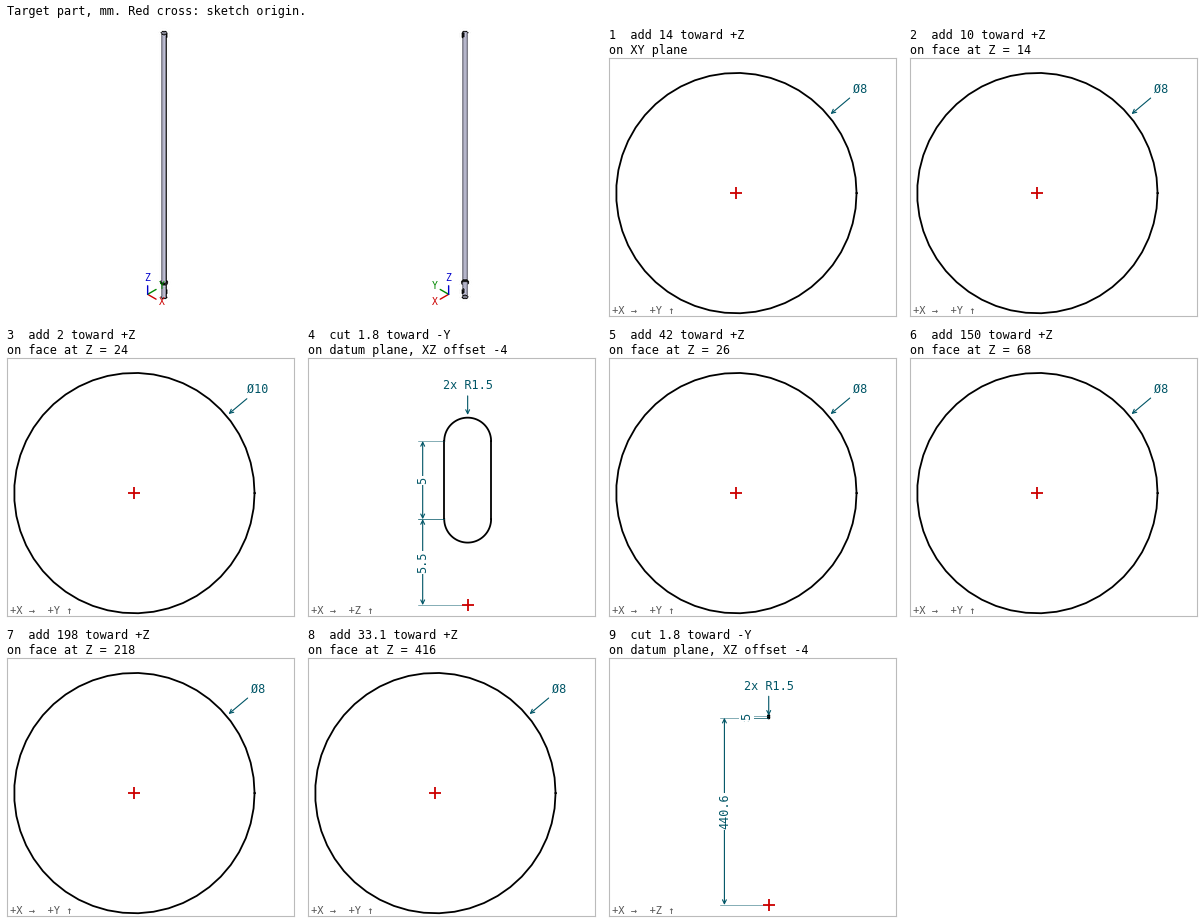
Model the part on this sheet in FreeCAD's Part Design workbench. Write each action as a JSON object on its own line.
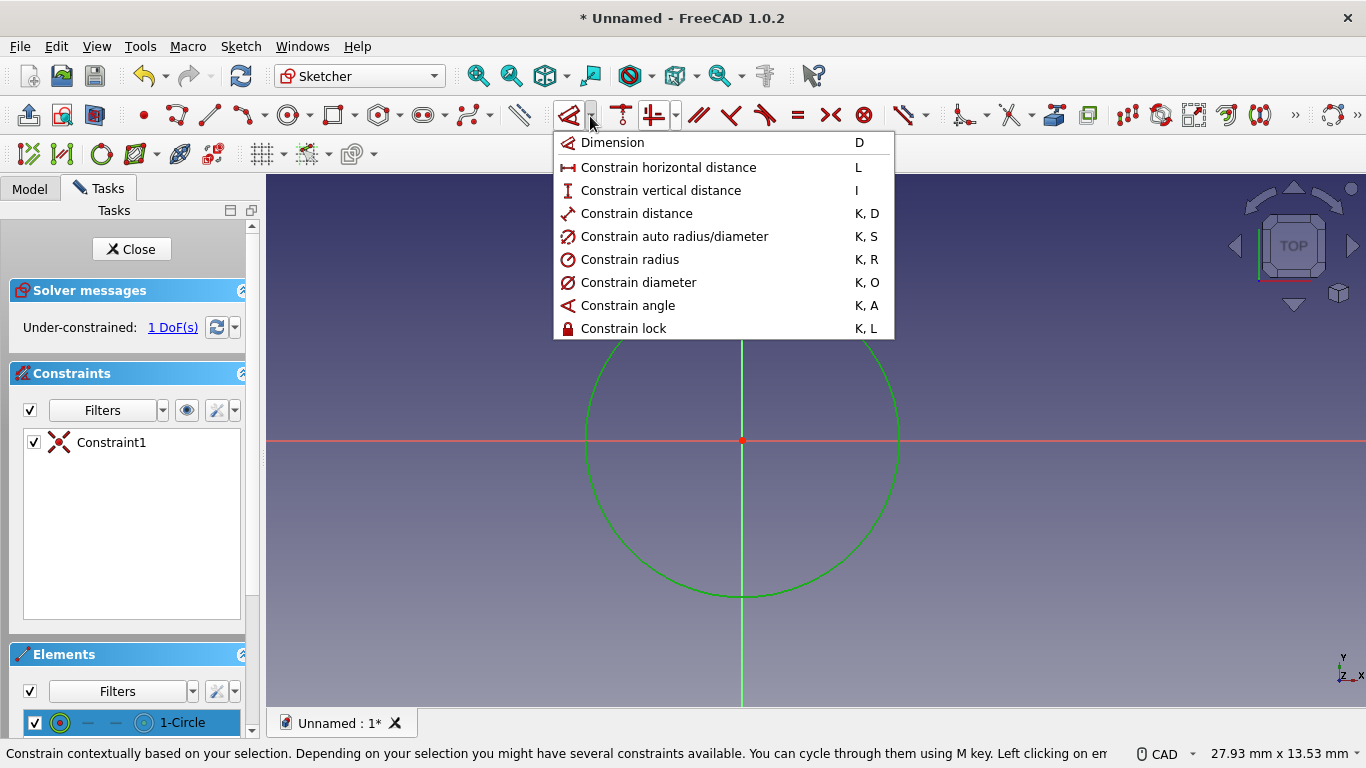
{"action": "left_click", "coordinate": [724, 282]}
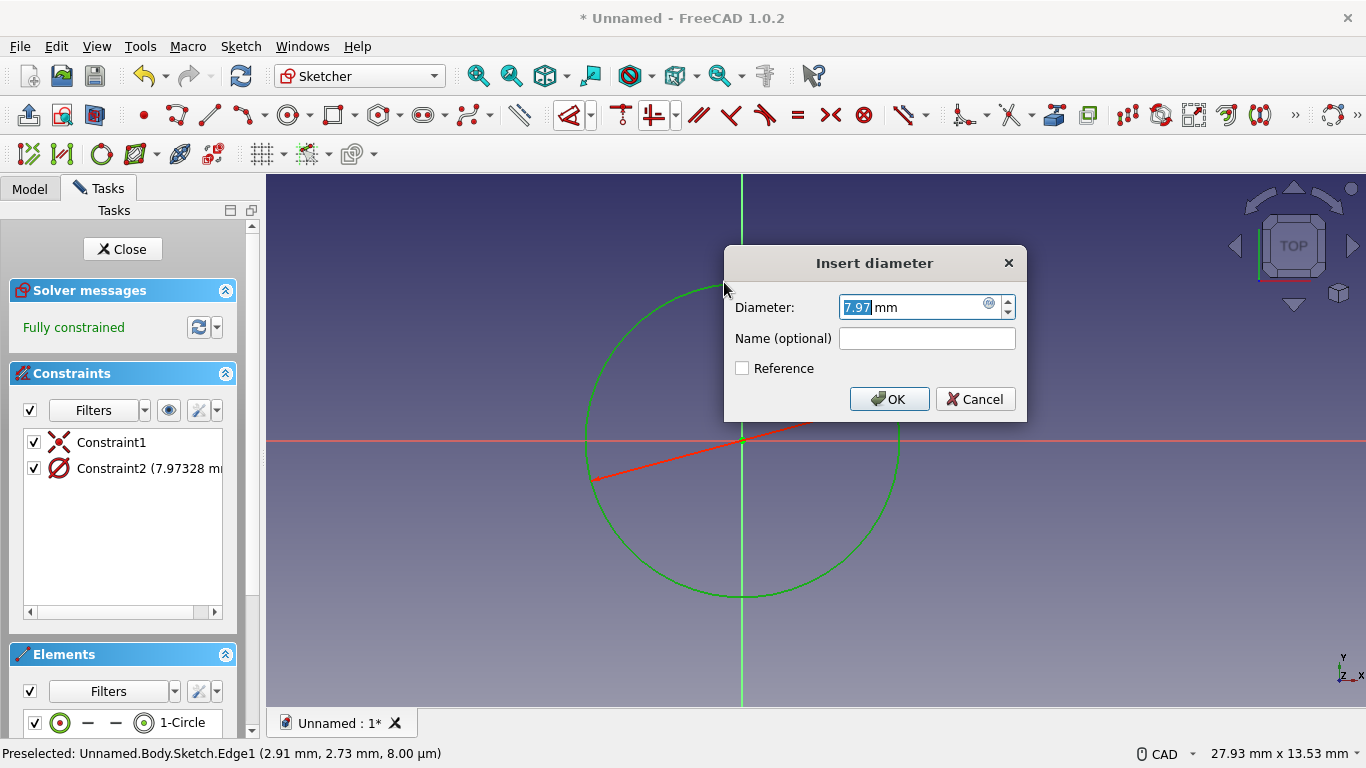
{"action": "type", "text": "8"}
{"action": "key", "text": "Return"}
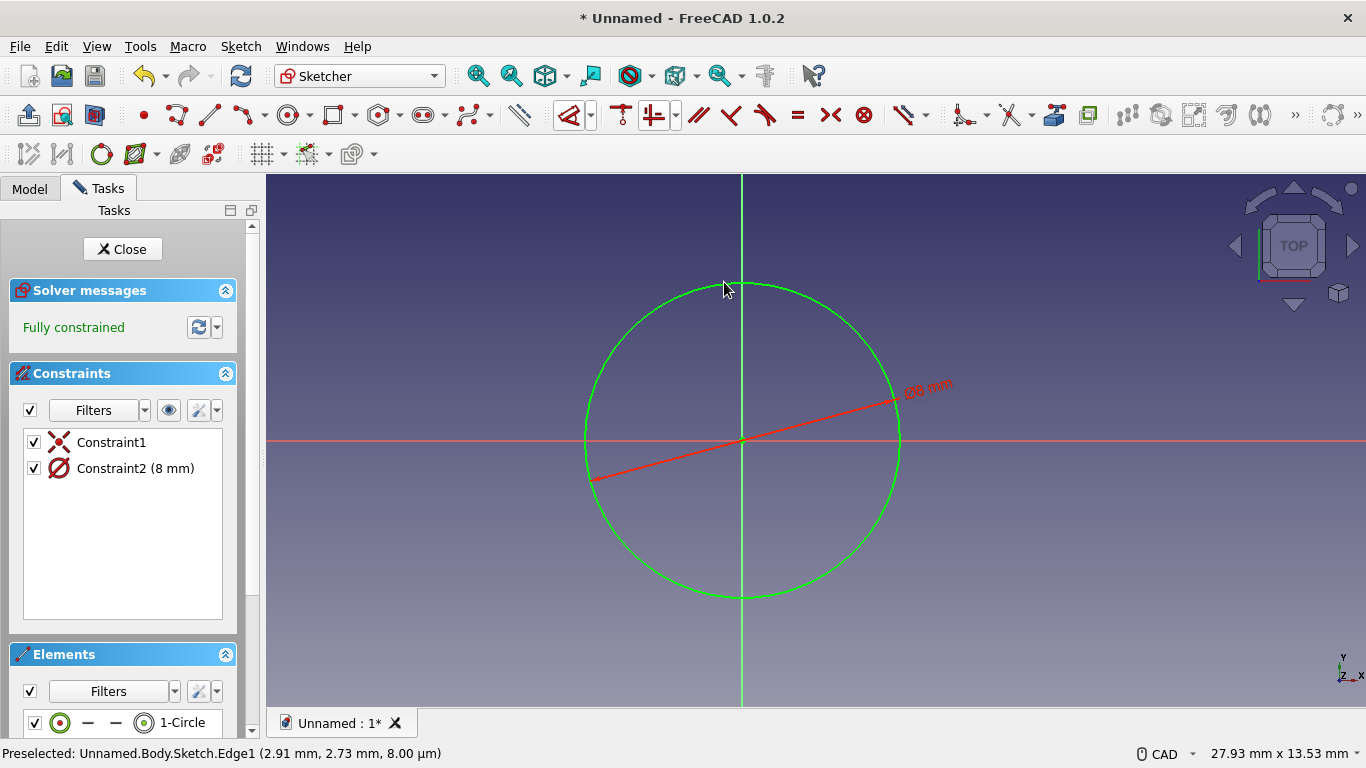
{"action": "left_click", "coordinate": [123, 249]}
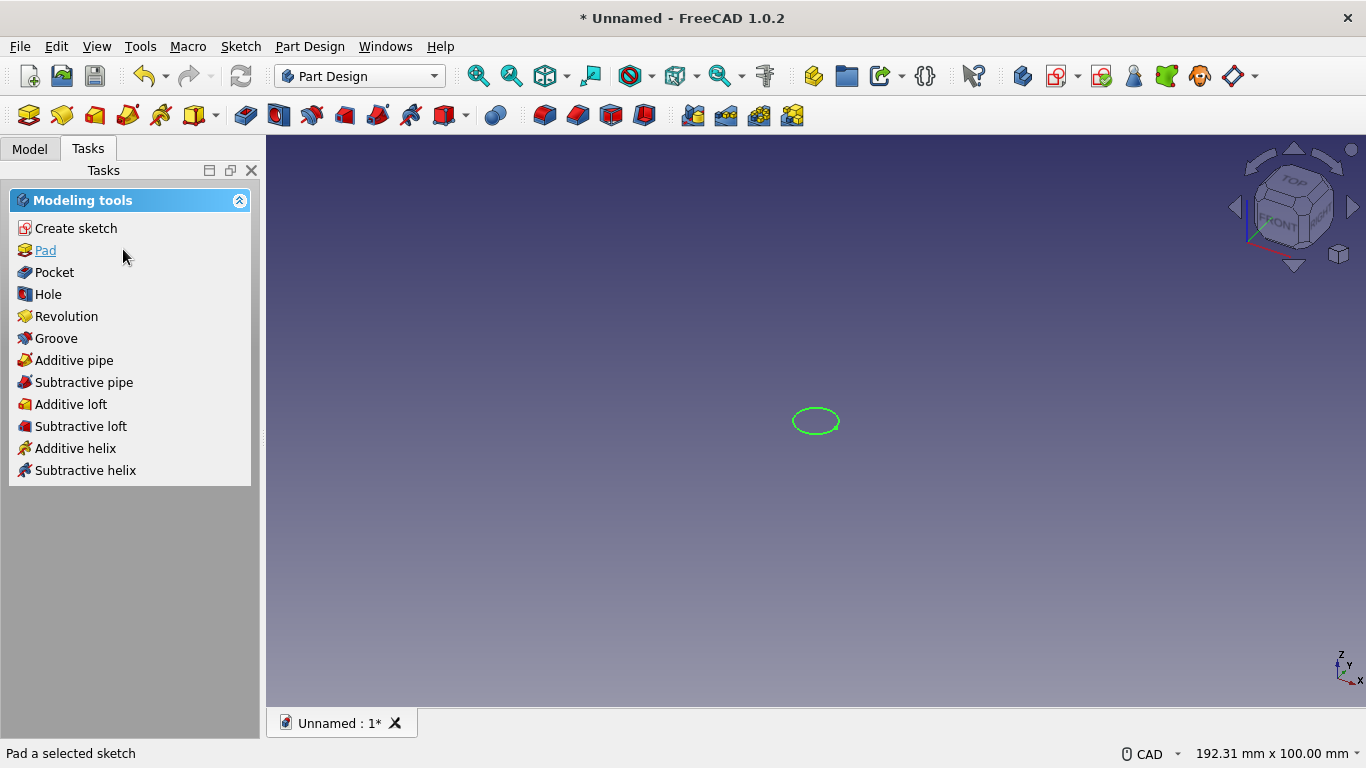
{"action": "left_click", "coordinate": [29, 116]}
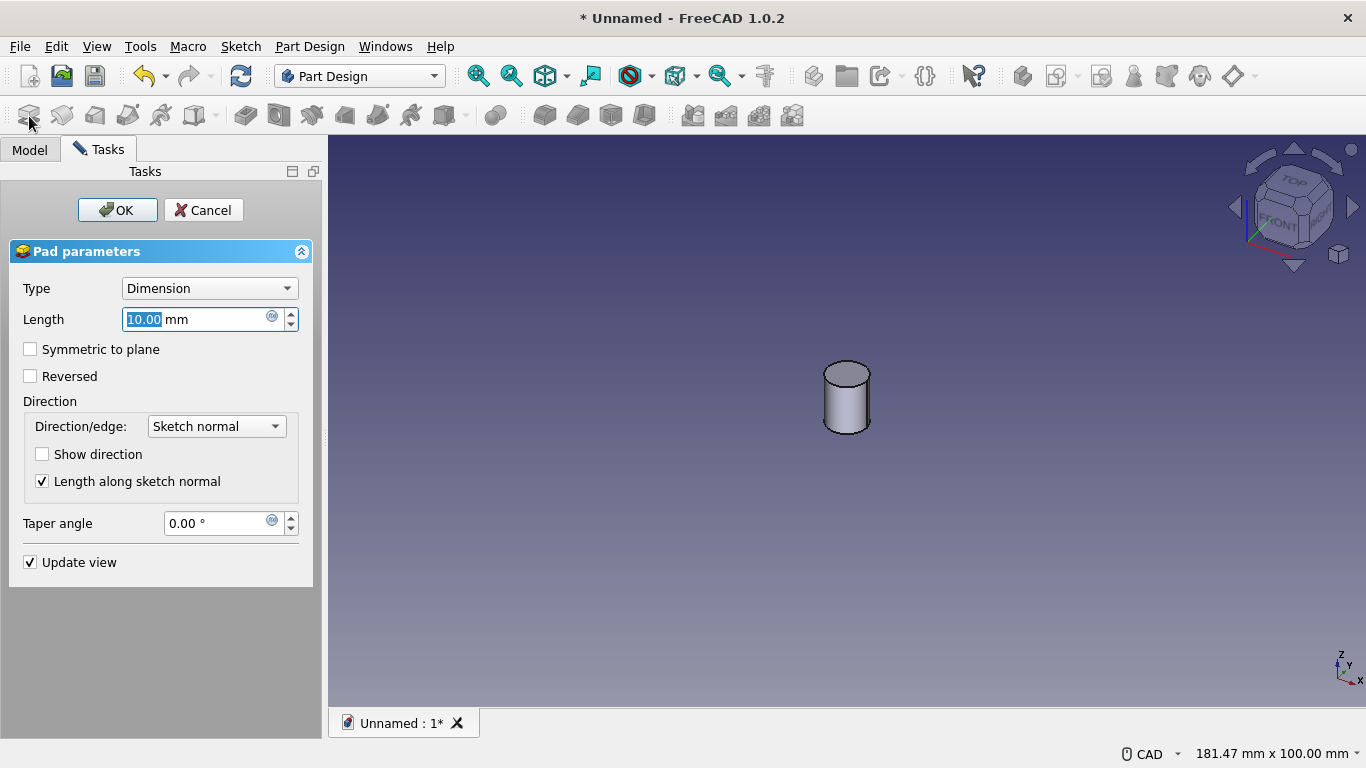
{"action": "type", "text": "14"}
{"action": "key", "text": "Tab"}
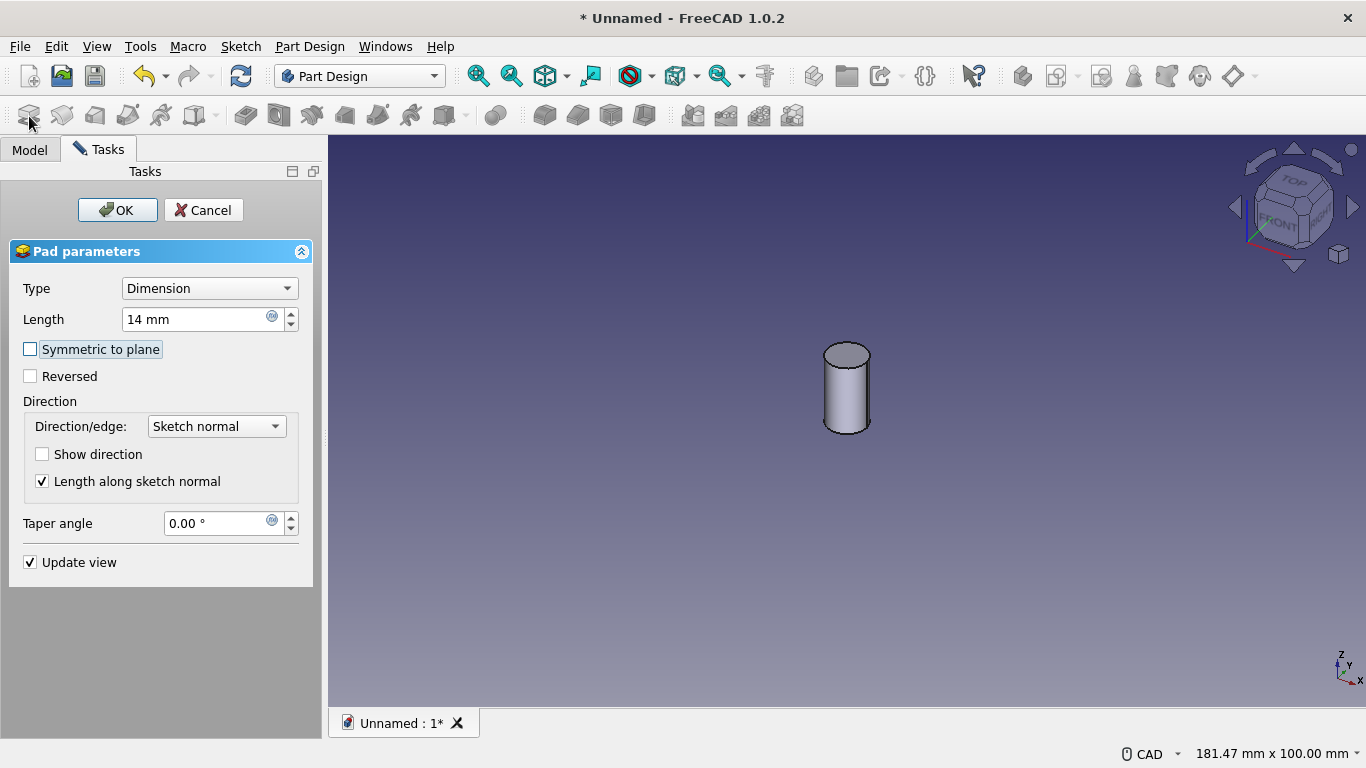
{"action": "left_click", "coordinate": [118, 210]}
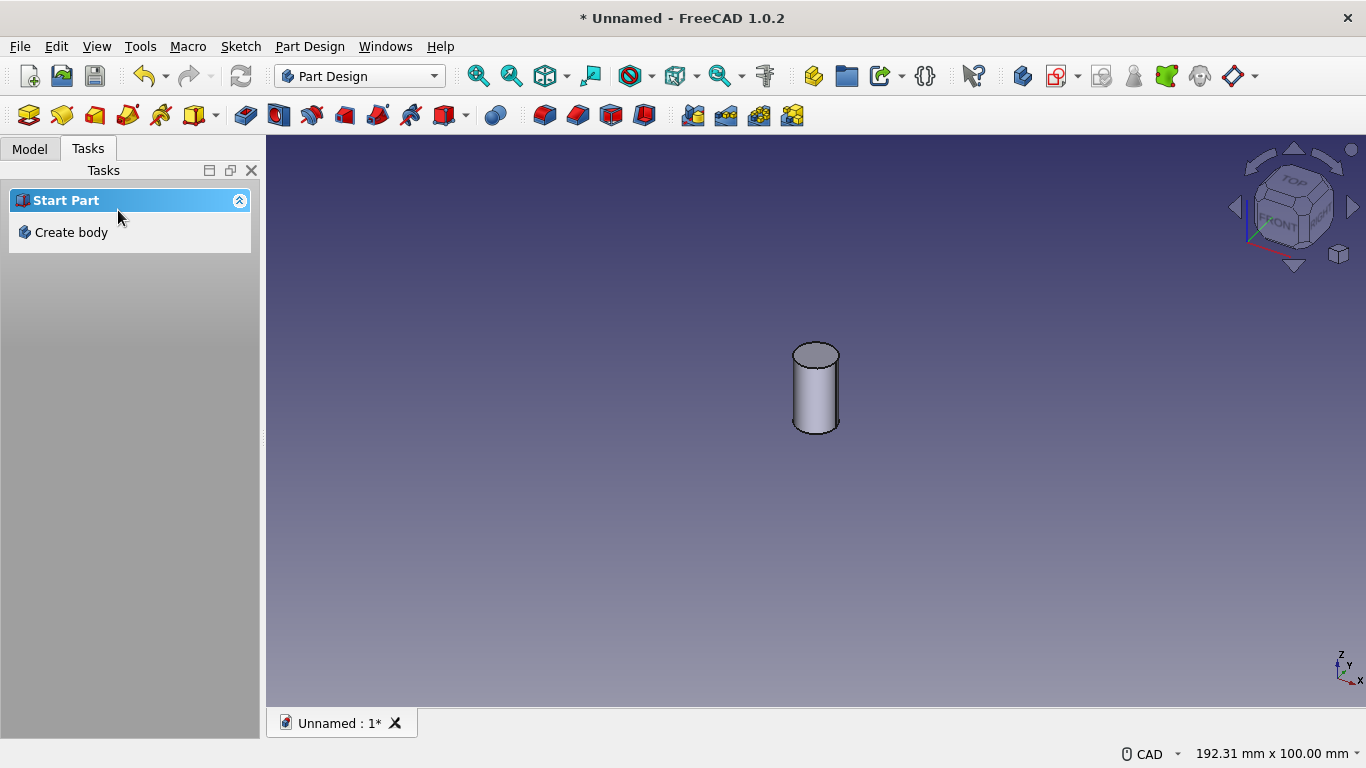
{"action": "left_click", "coordinate": [479, 76]}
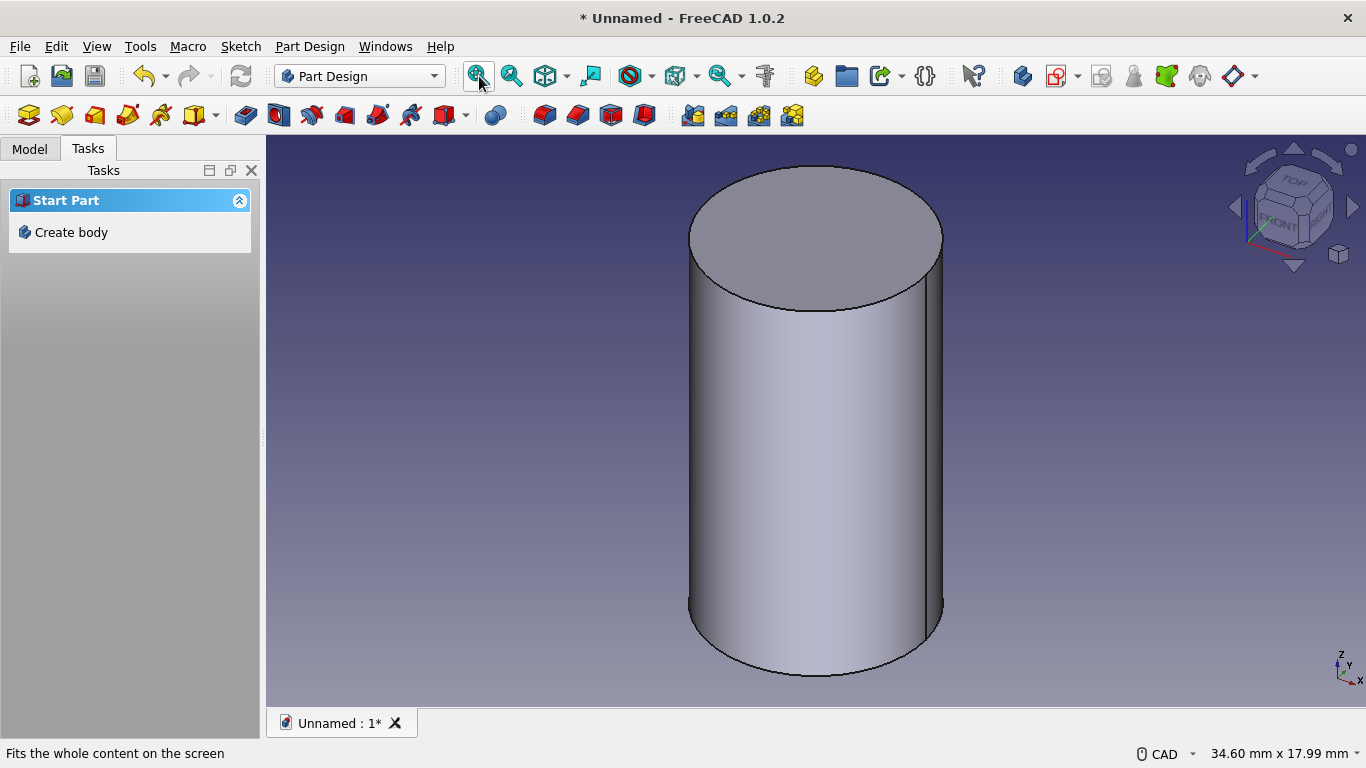
{"action": "left_click", "coordinate": [816, 238]}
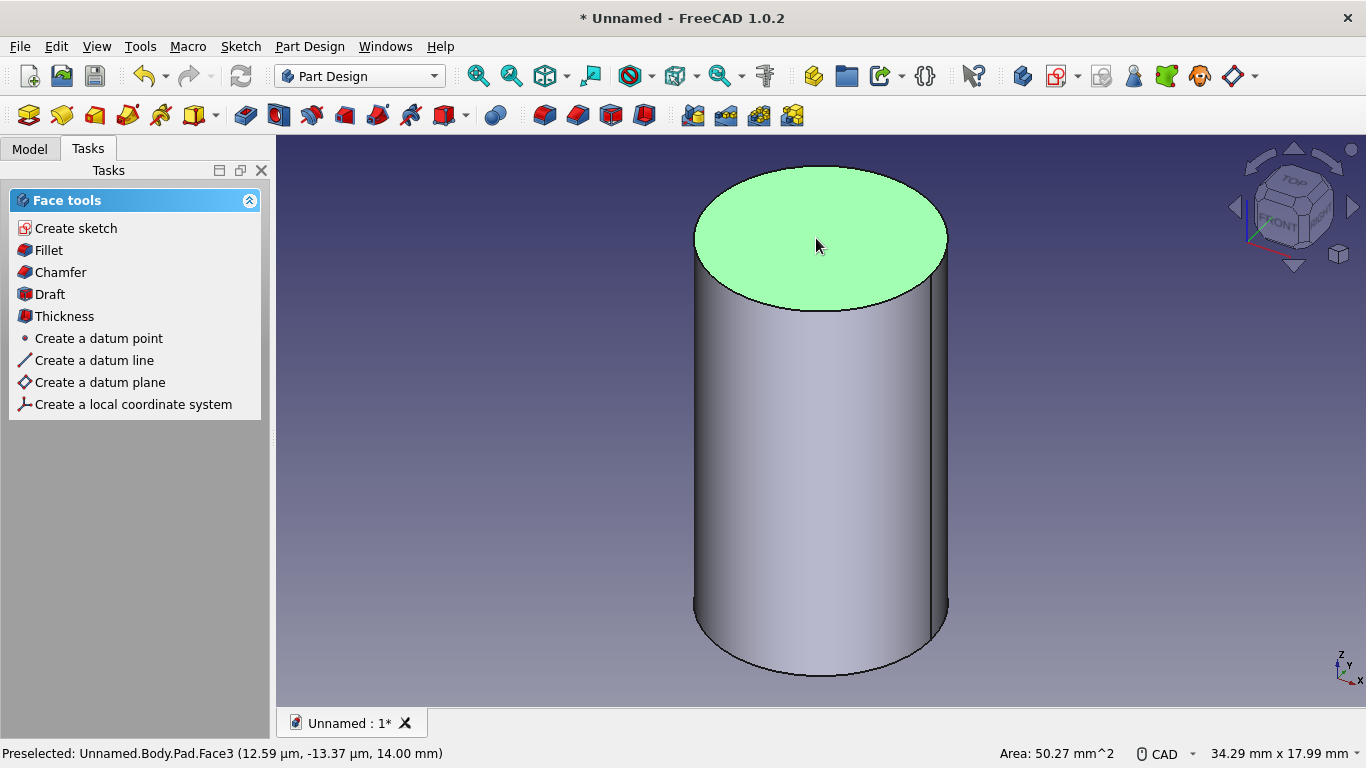
{"action": "left_click", "coordinate": [1056, 76]}